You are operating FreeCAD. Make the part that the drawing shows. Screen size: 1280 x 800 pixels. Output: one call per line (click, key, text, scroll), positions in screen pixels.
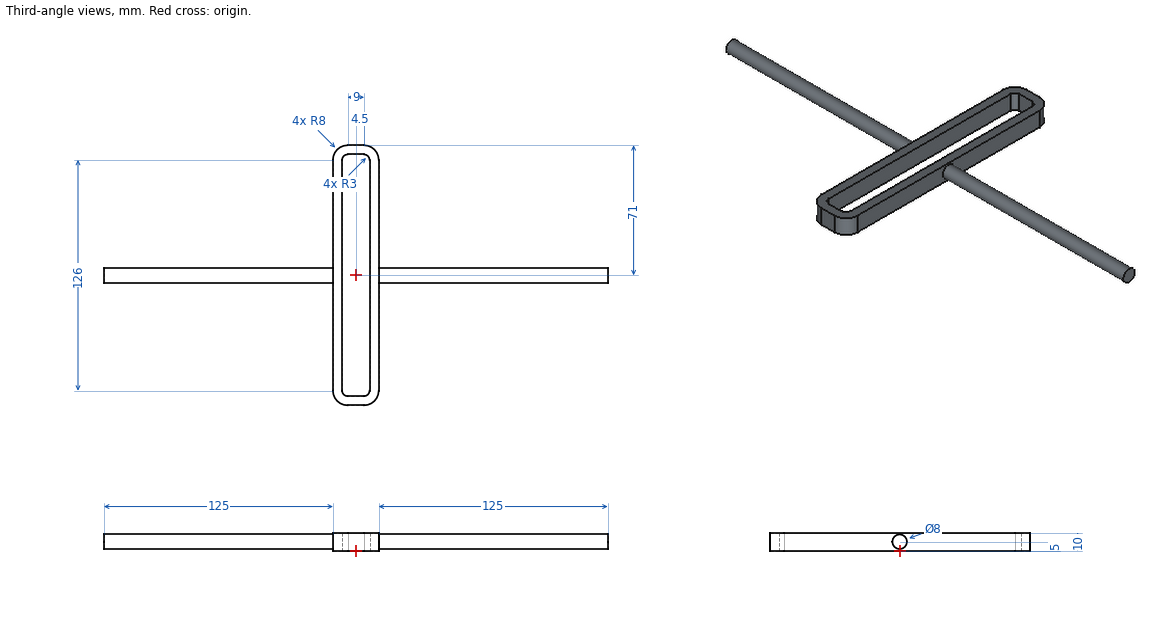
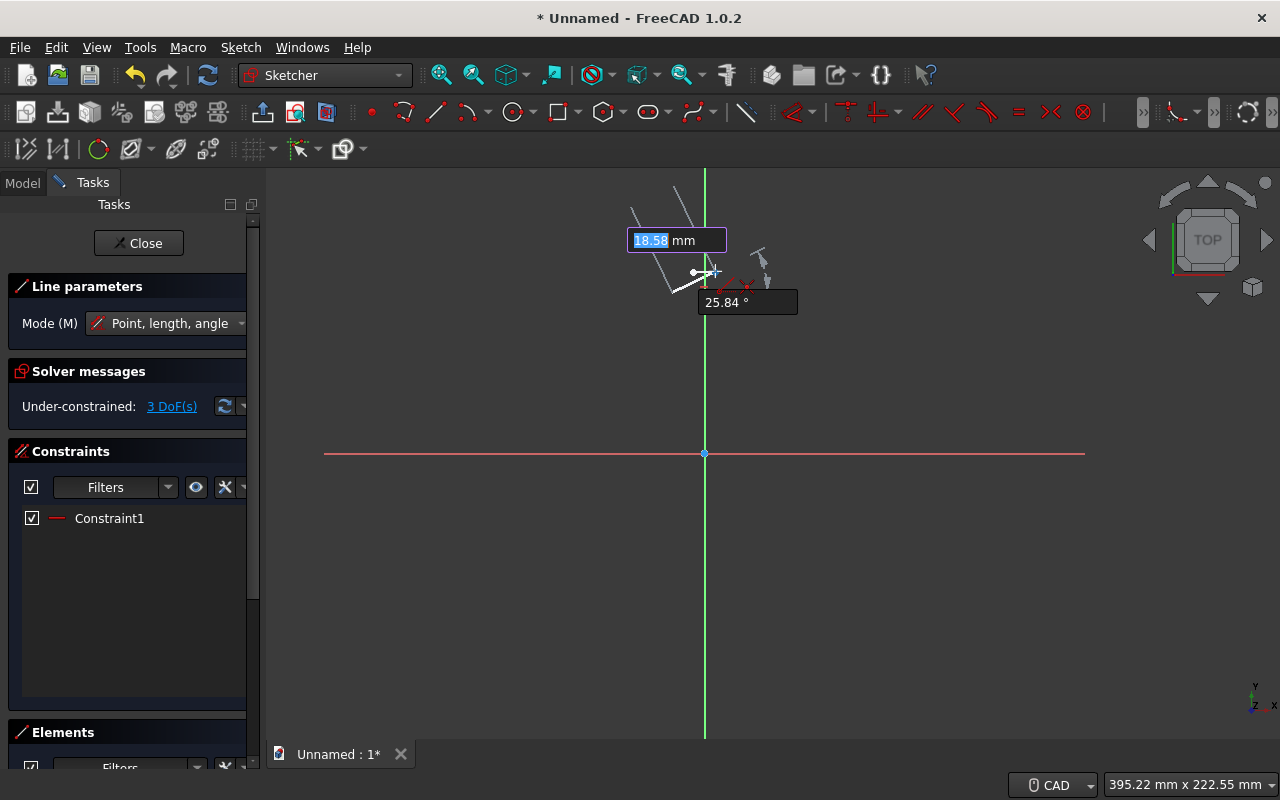
click(672, 615)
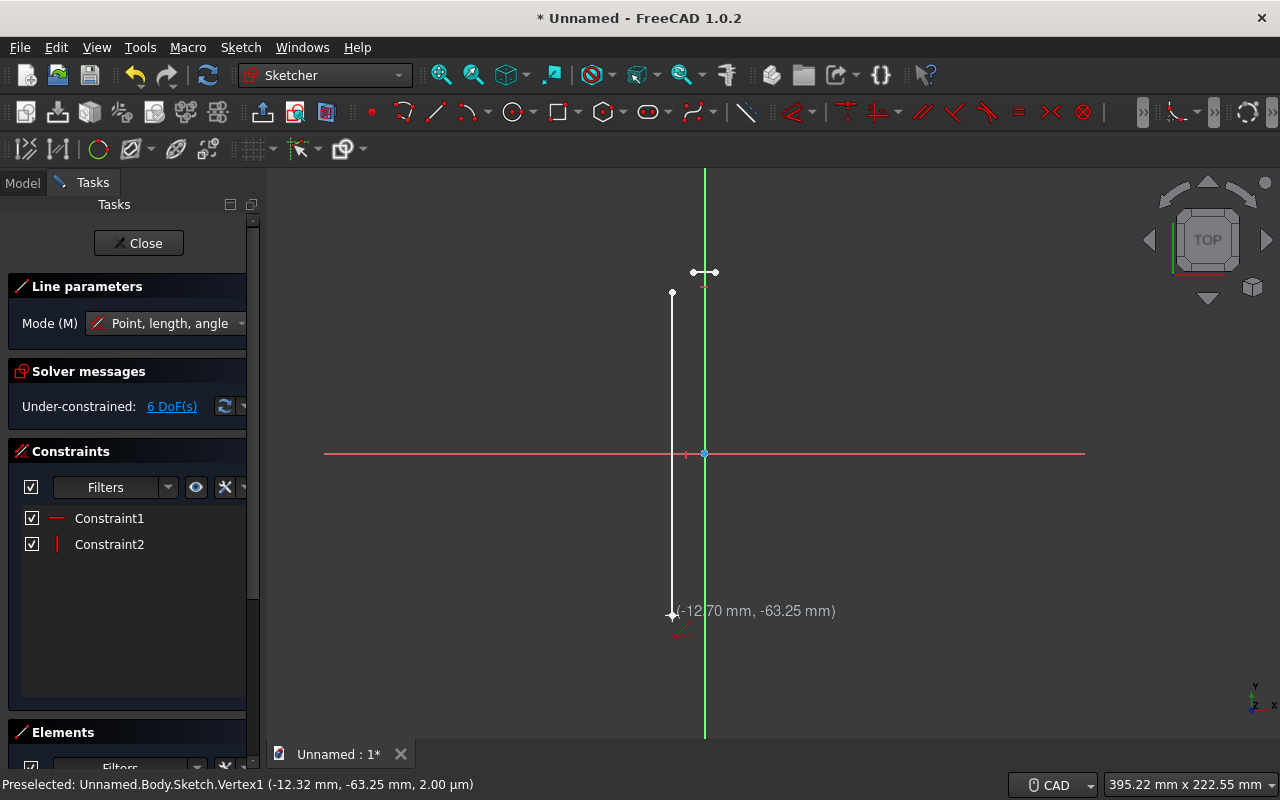
scroll(693, 636, up, 2)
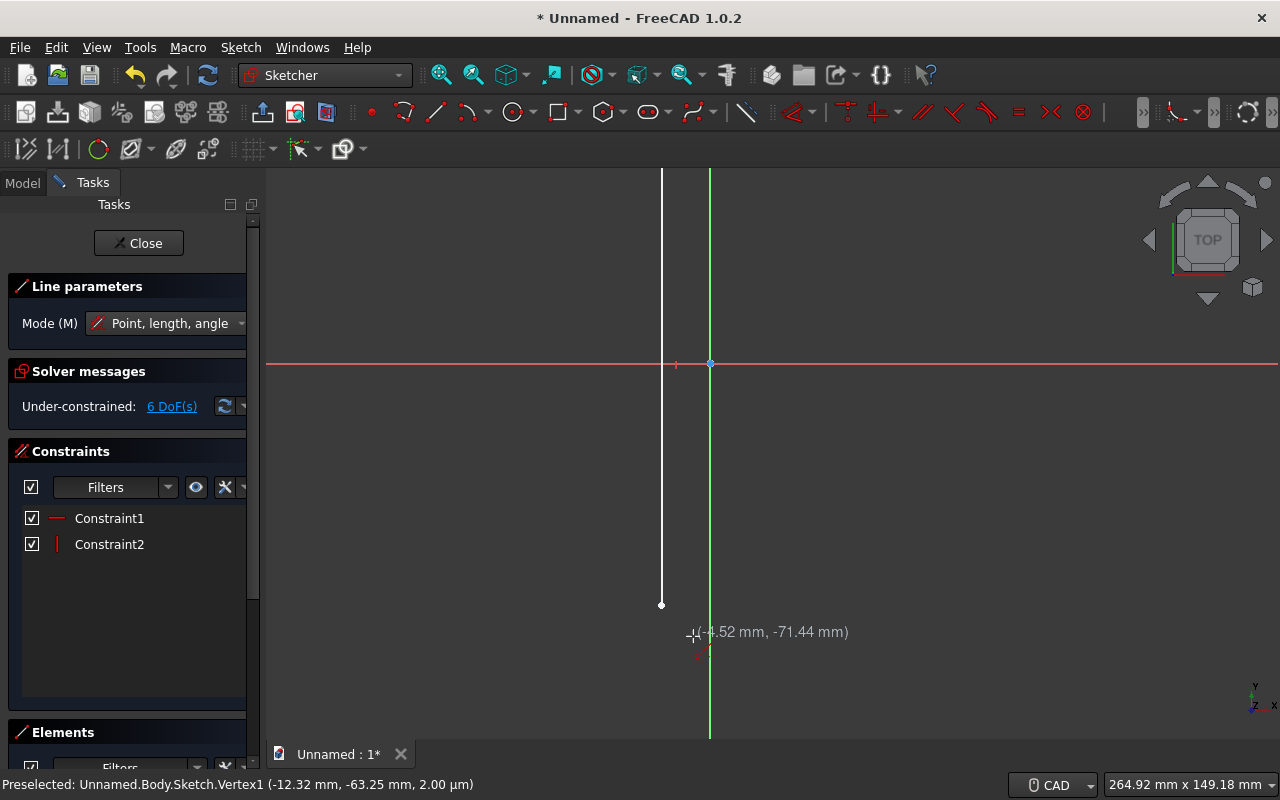
click(693, 635)
click(727, 635)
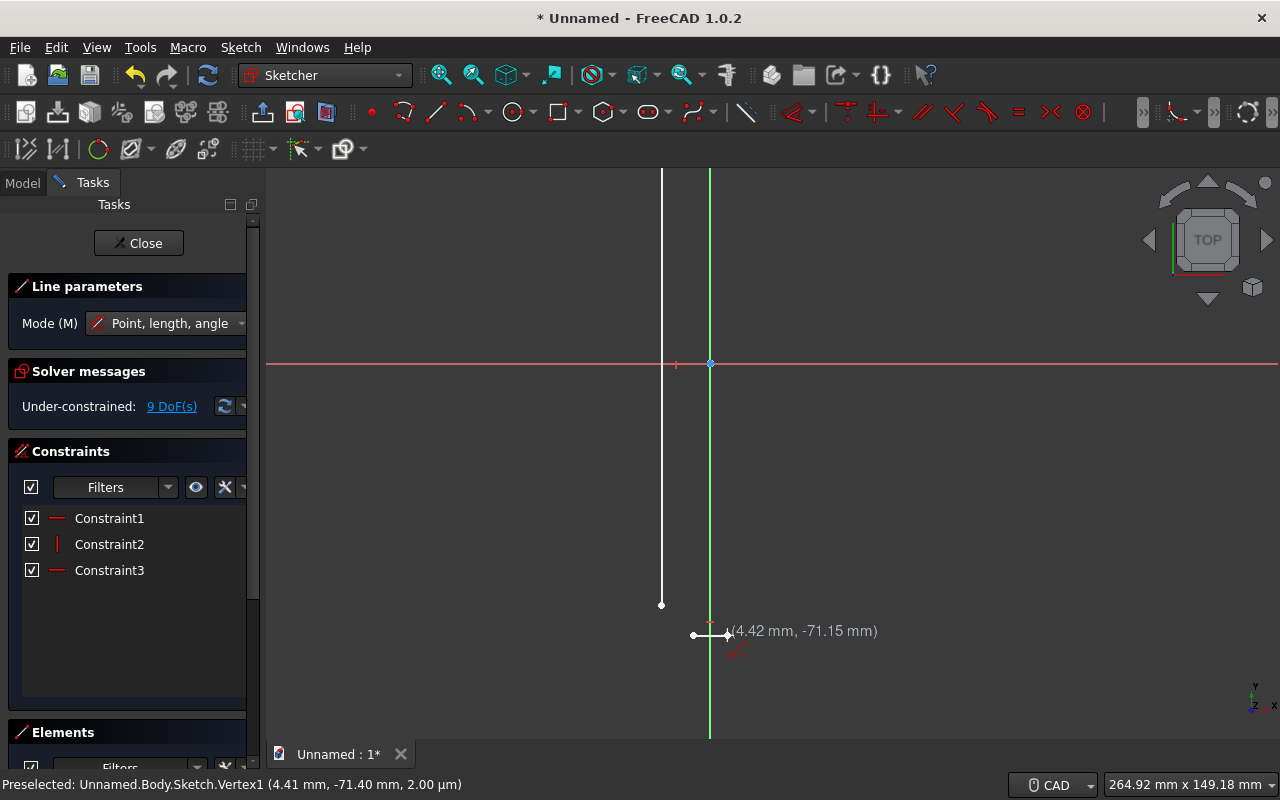
click(758, 605)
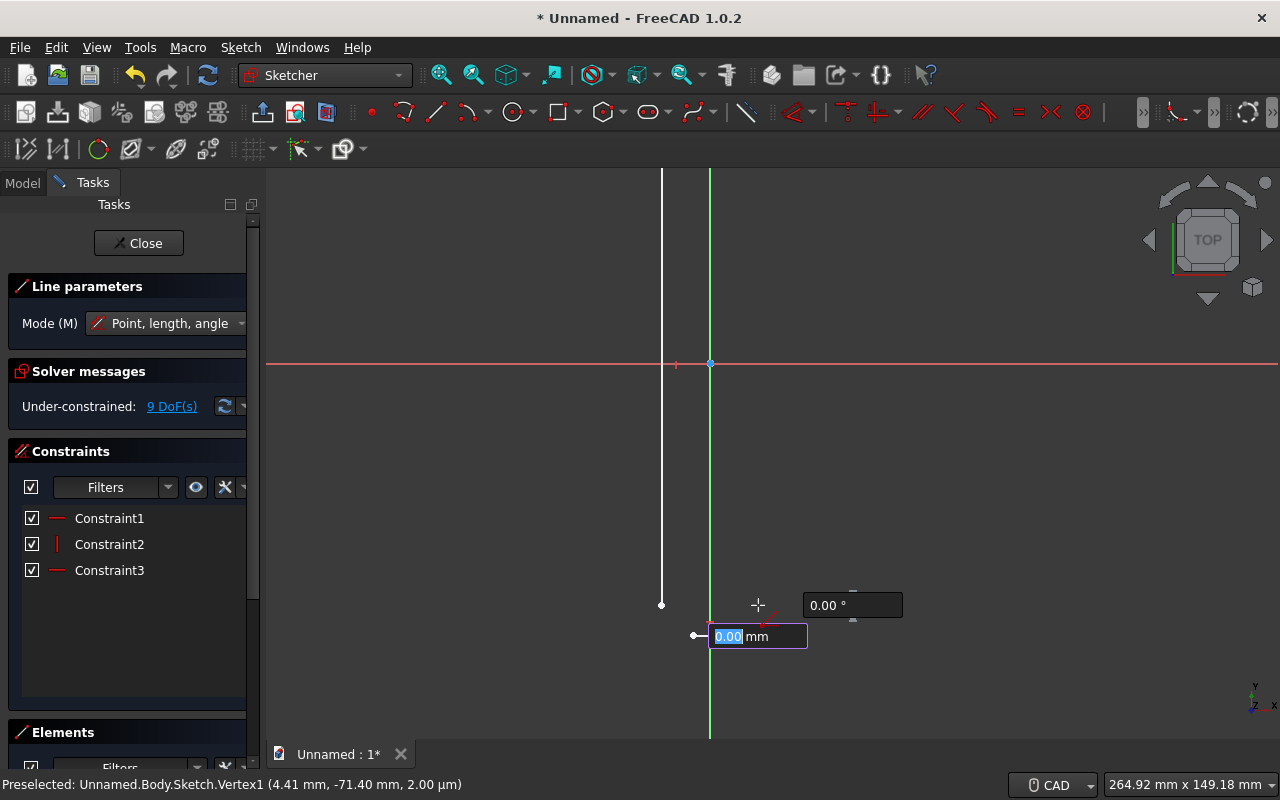
scroll(693, 636, down, 2)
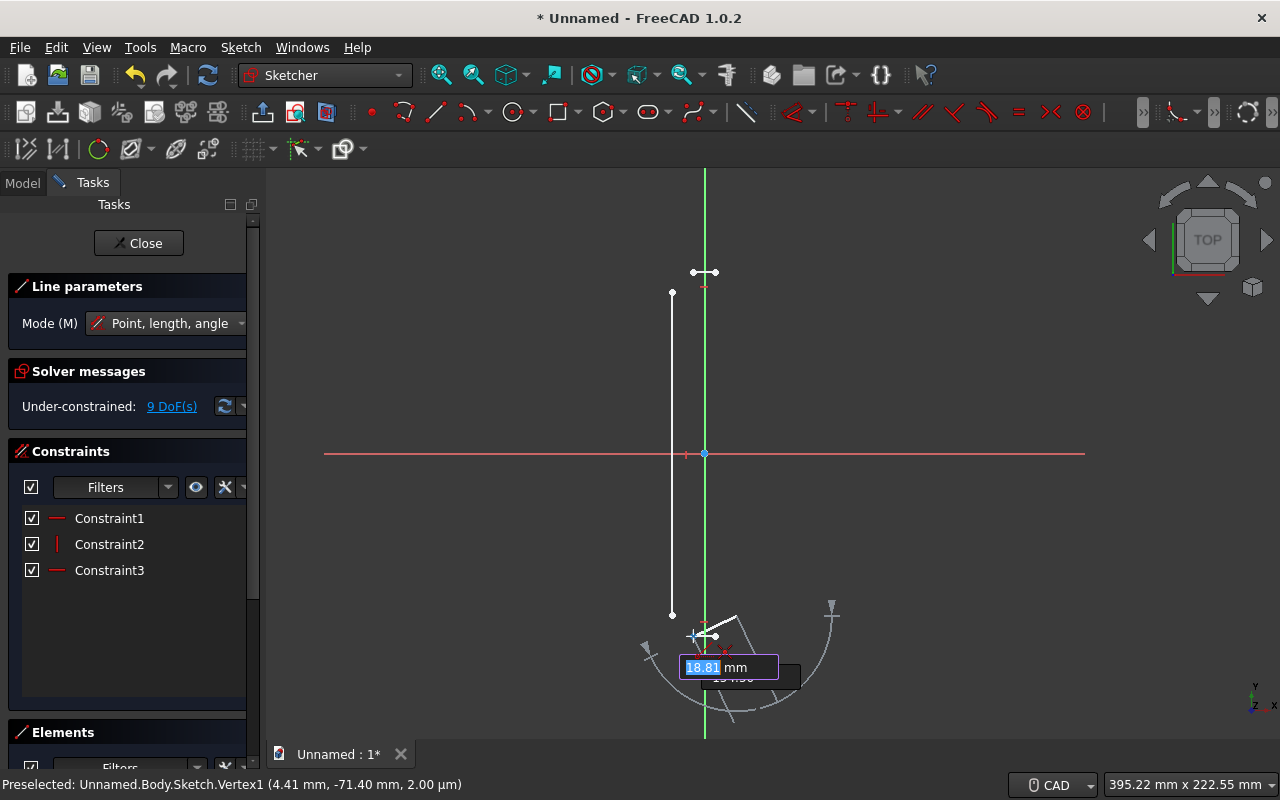
click(737, 292)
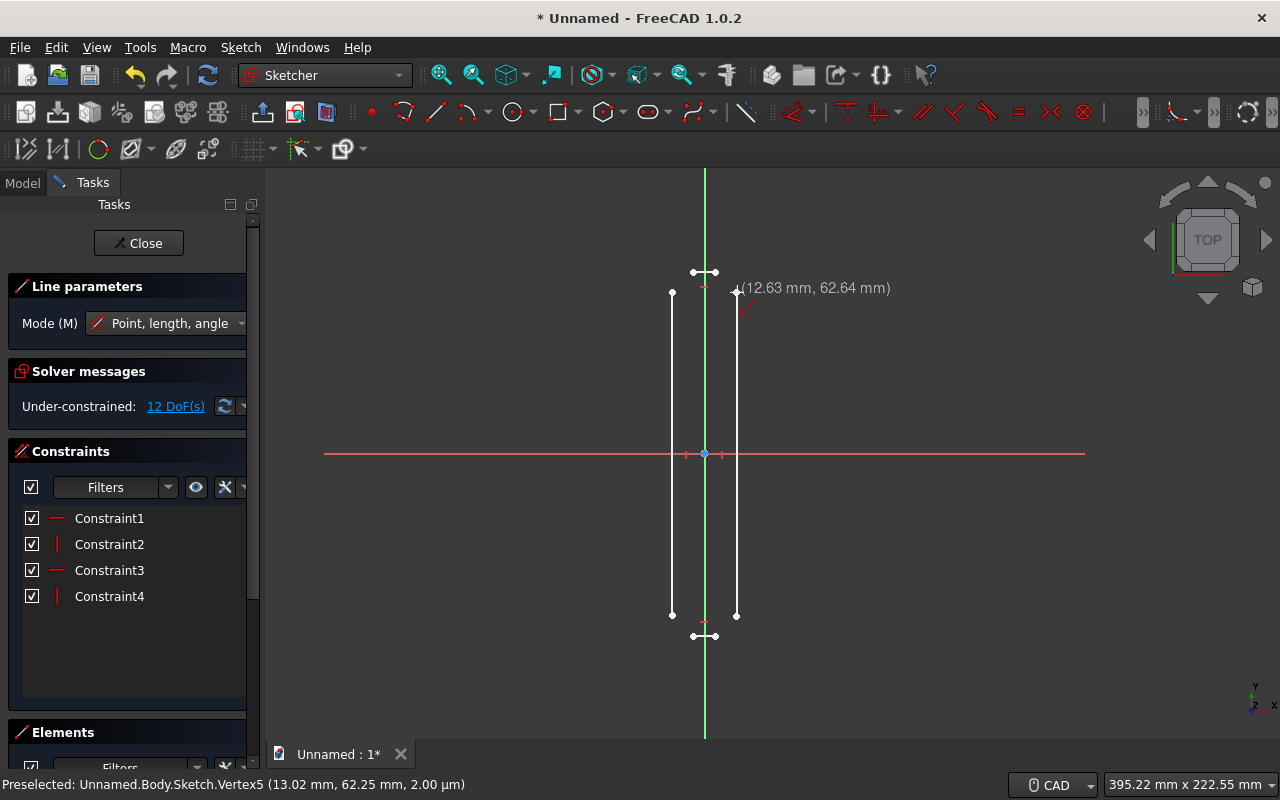
key(g)
key(3)
key(a)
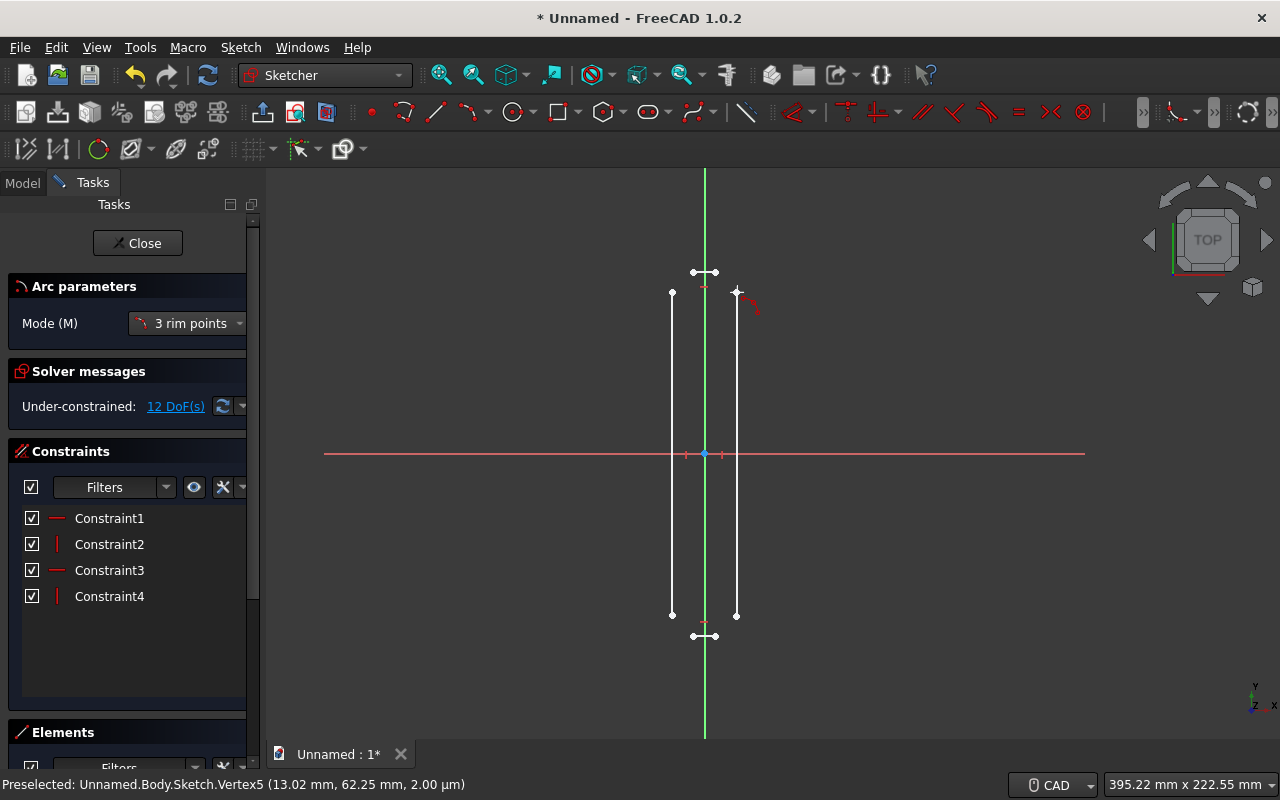
scroll(693, 272, up, 2)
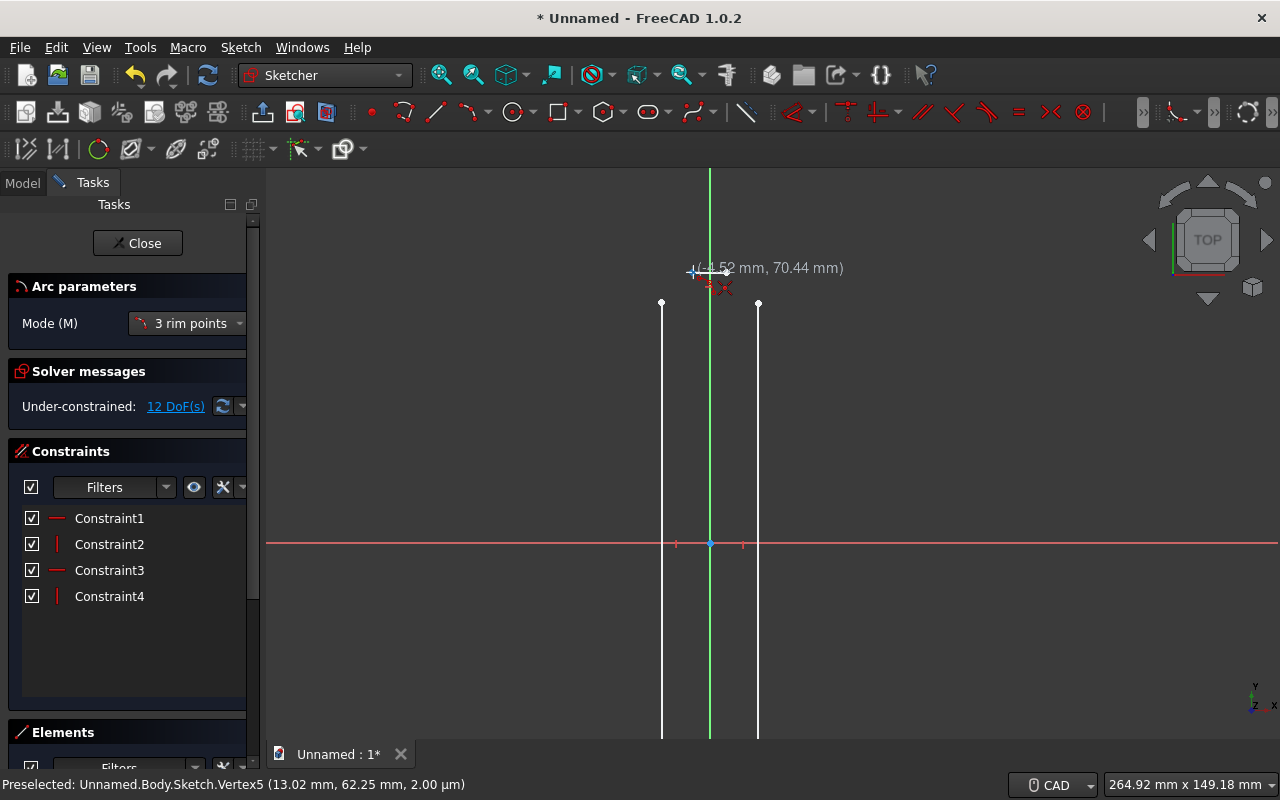
click(693, 273)
click(662, 303)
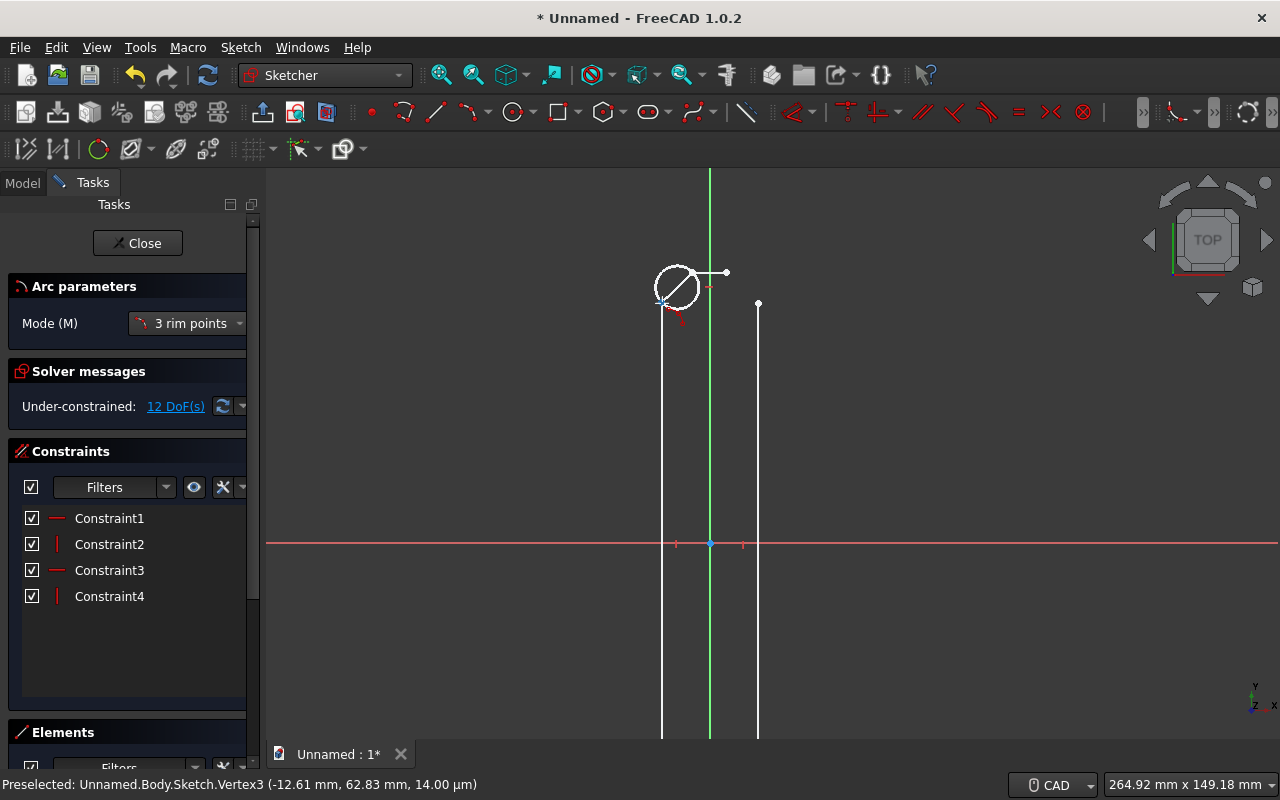
scroll(671, 280, up, 3)